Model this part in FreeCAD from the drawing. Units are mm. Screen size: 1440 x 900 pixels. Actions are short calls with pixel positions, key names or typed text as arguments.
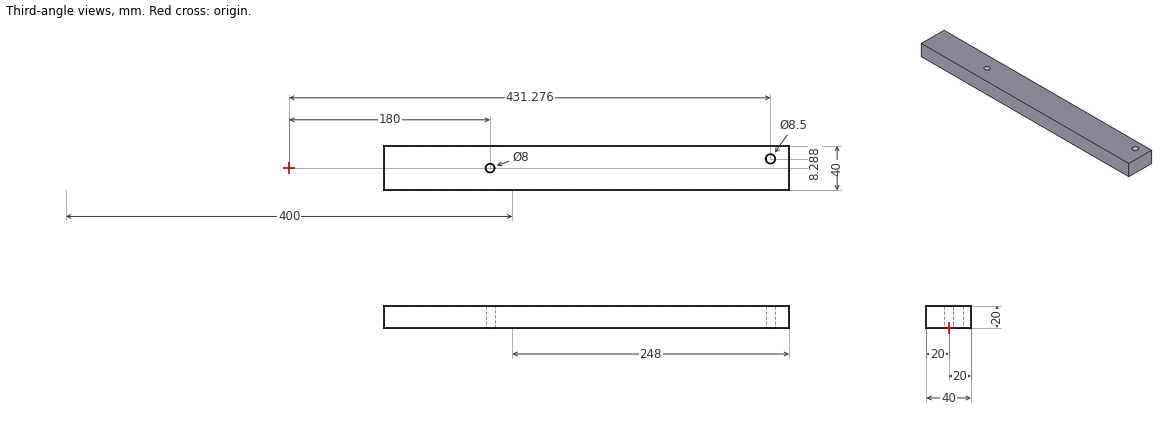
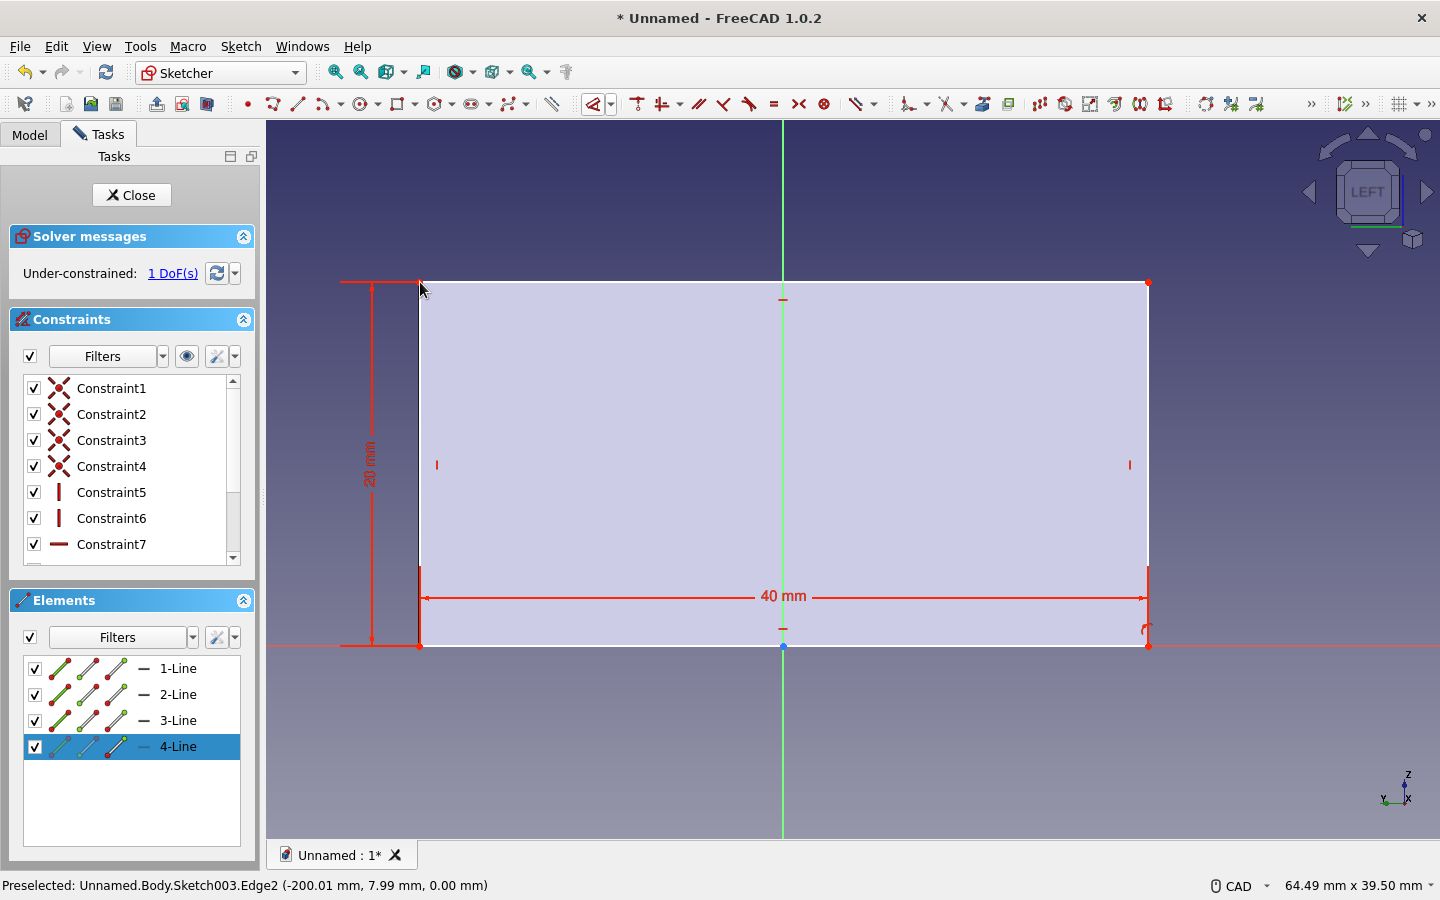
click(610, 104)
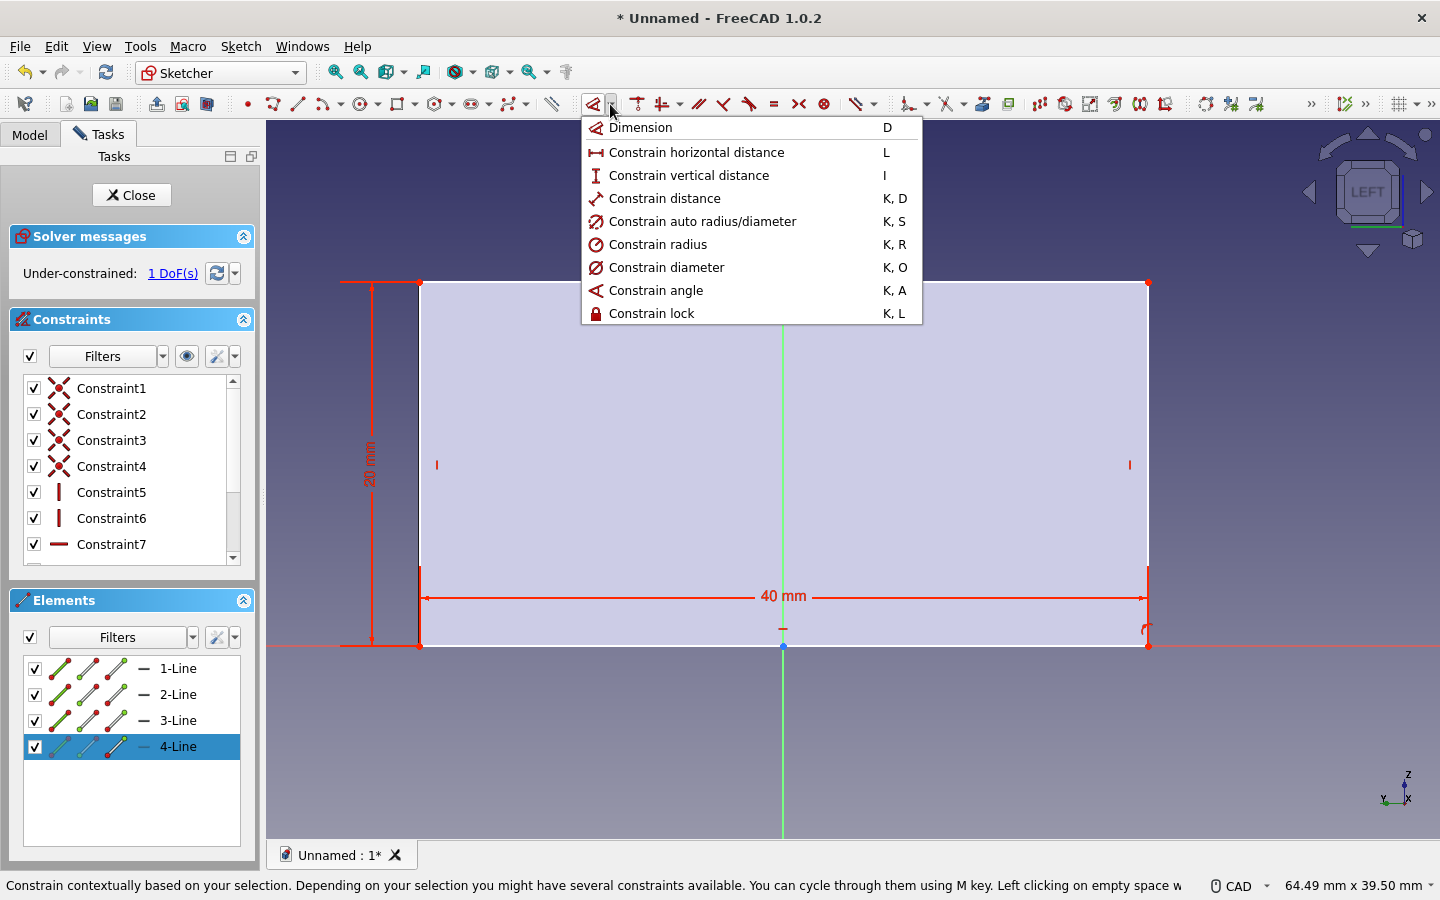
click(752, 152)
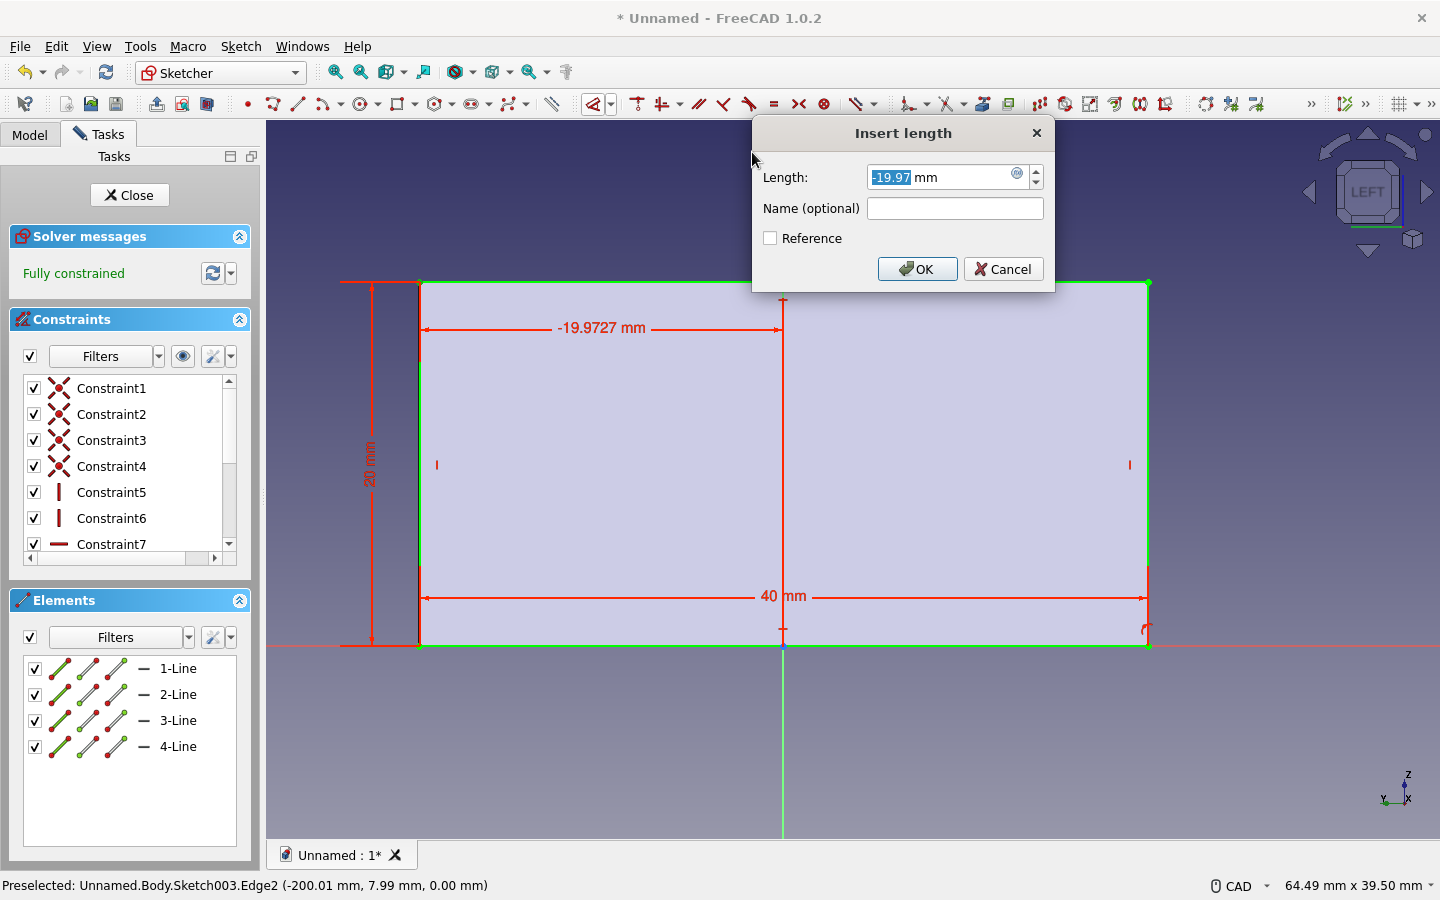
text(-20)
key(Return)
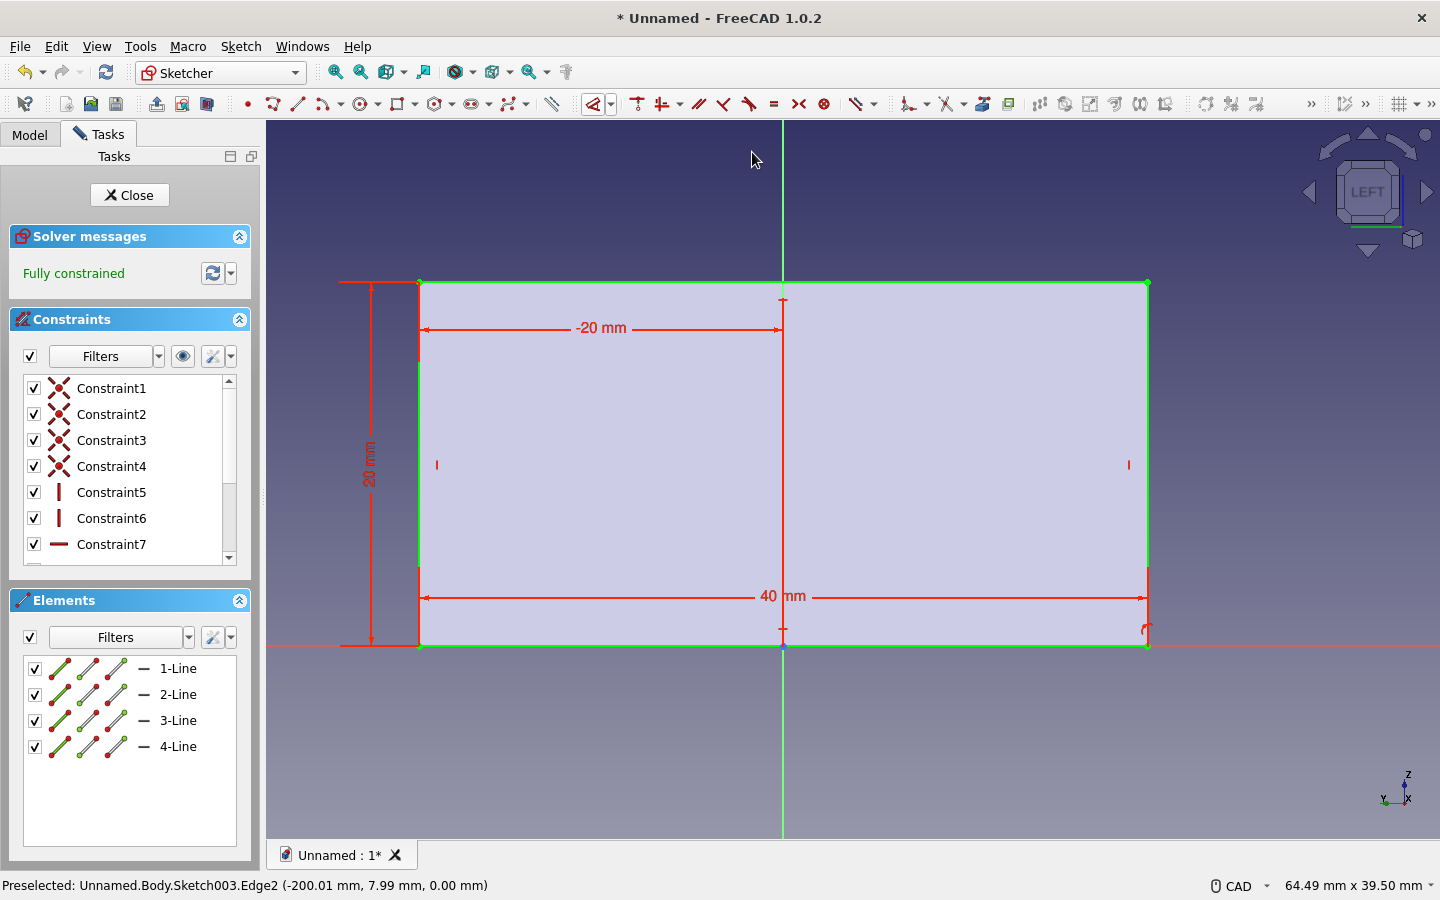
click(130, 195)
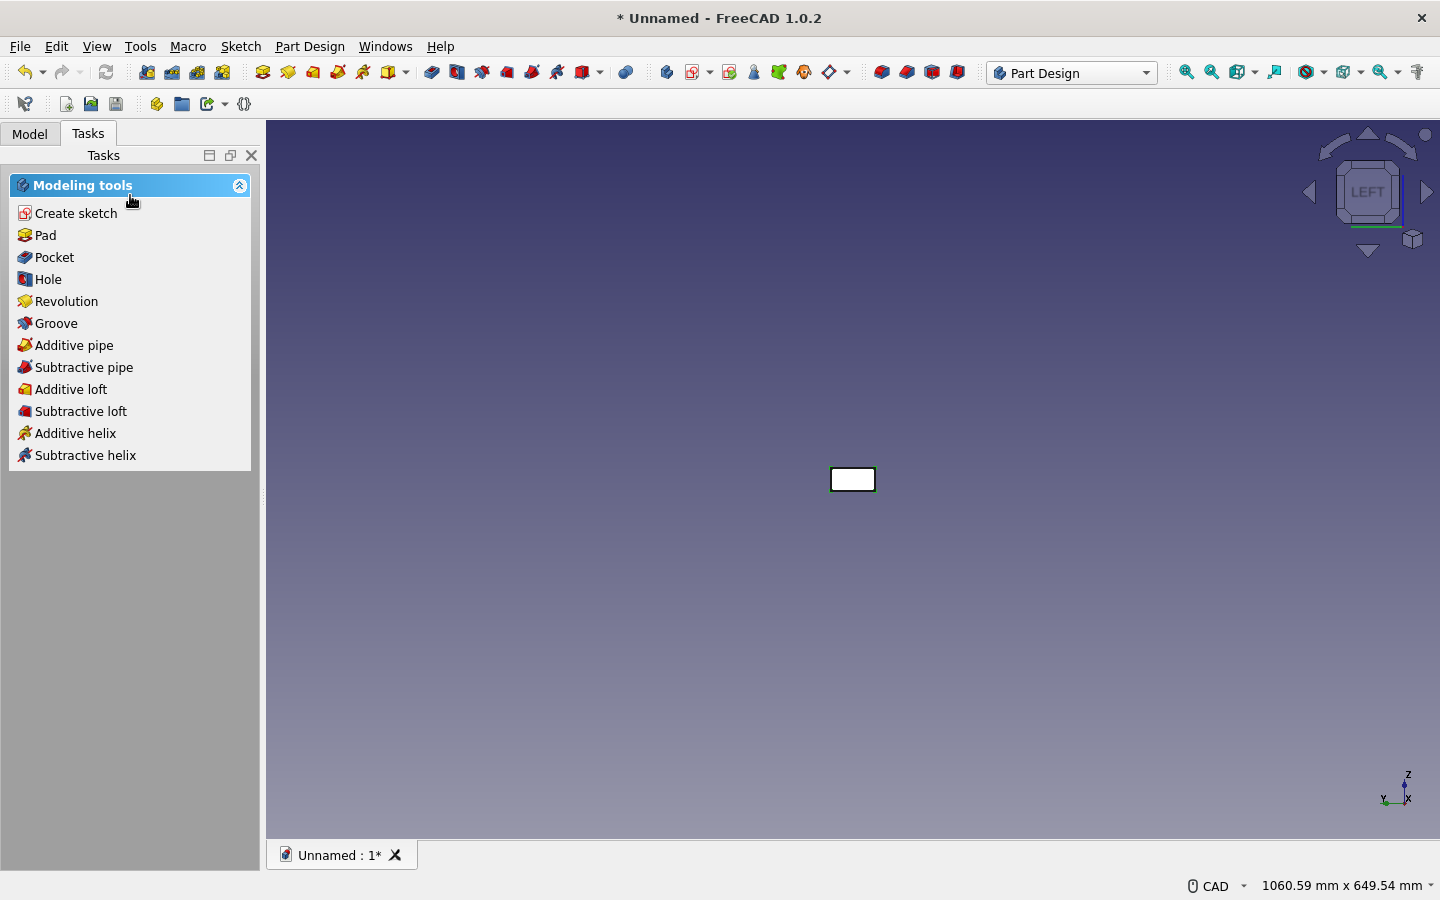
click(432, 72)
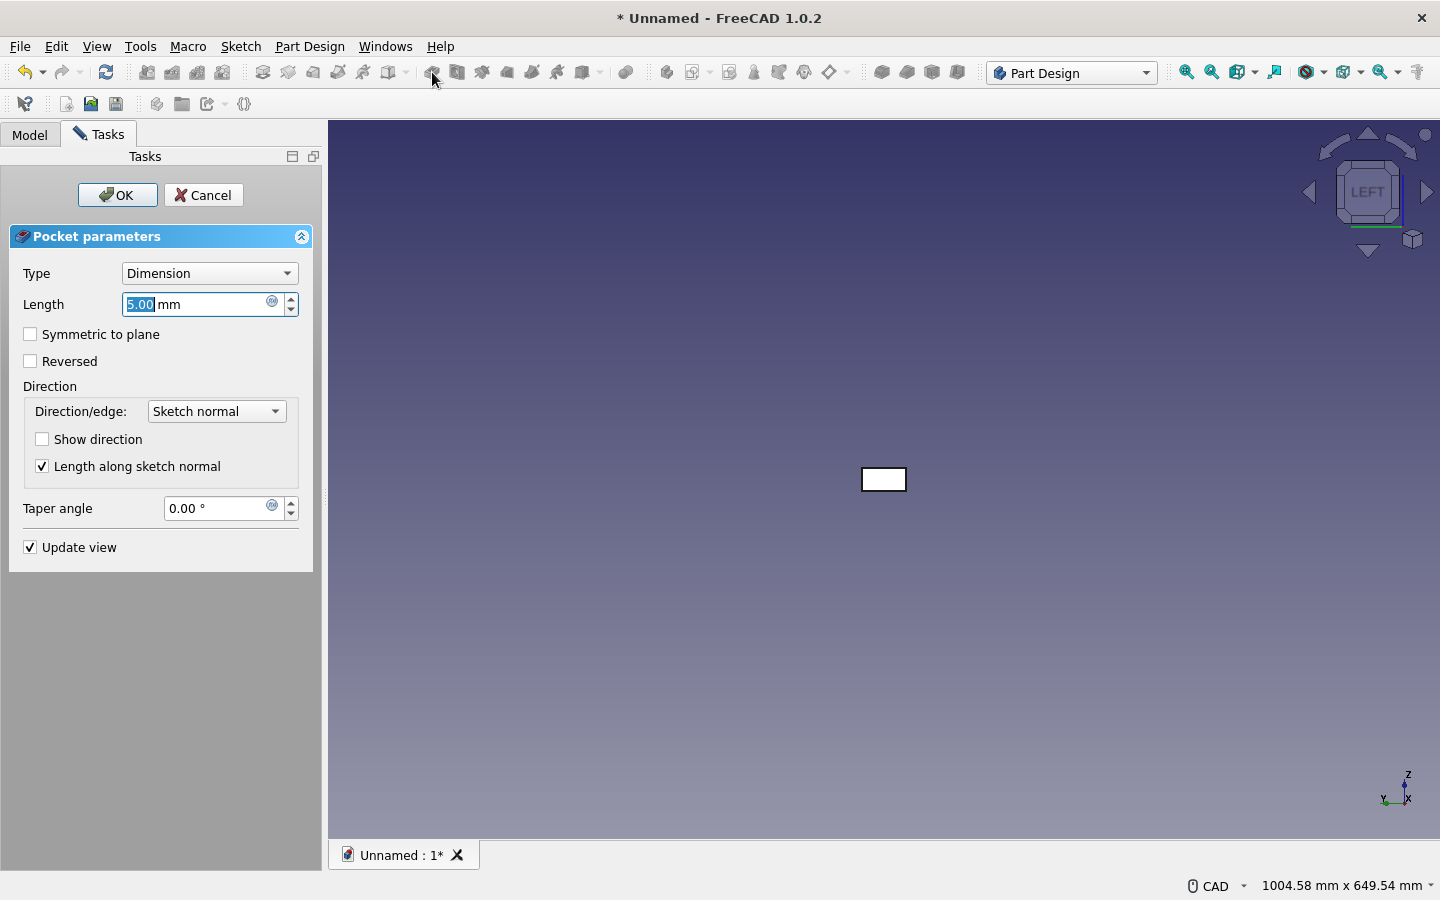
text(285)
key(Tab)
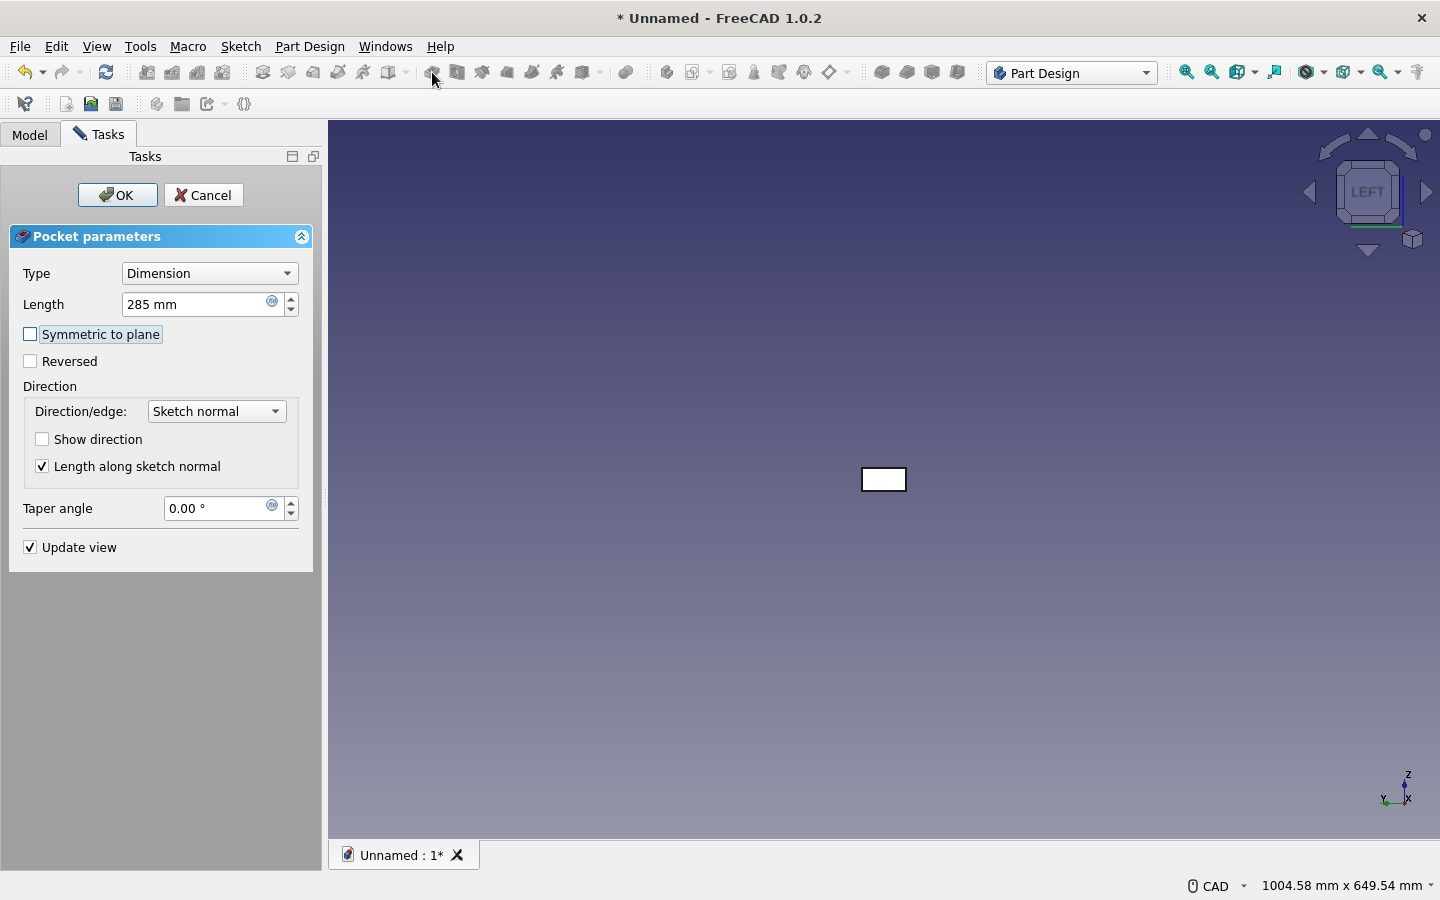
click(118, 195)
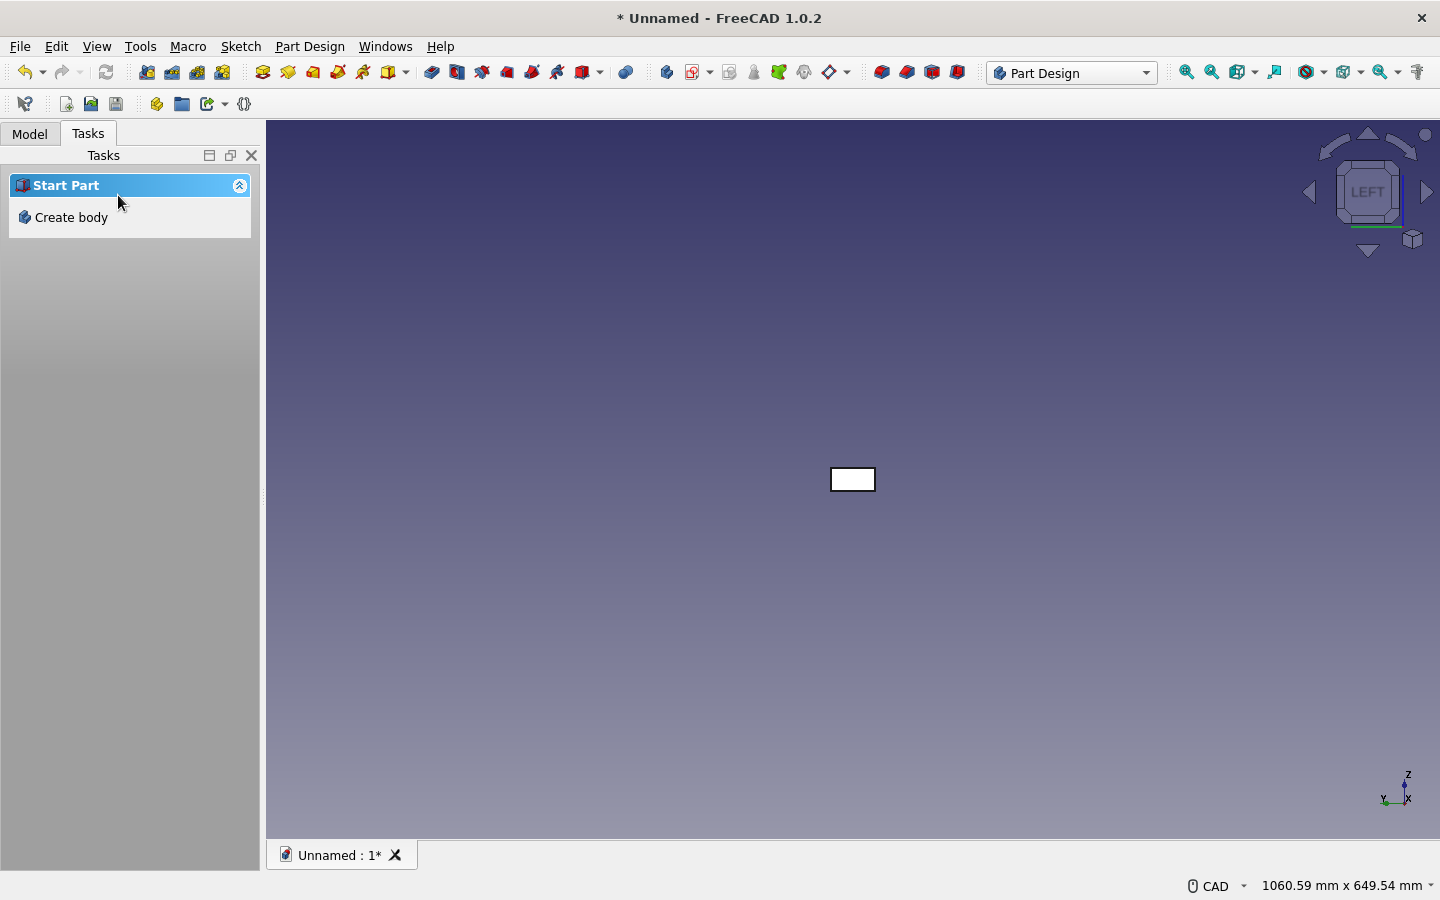
key(0)